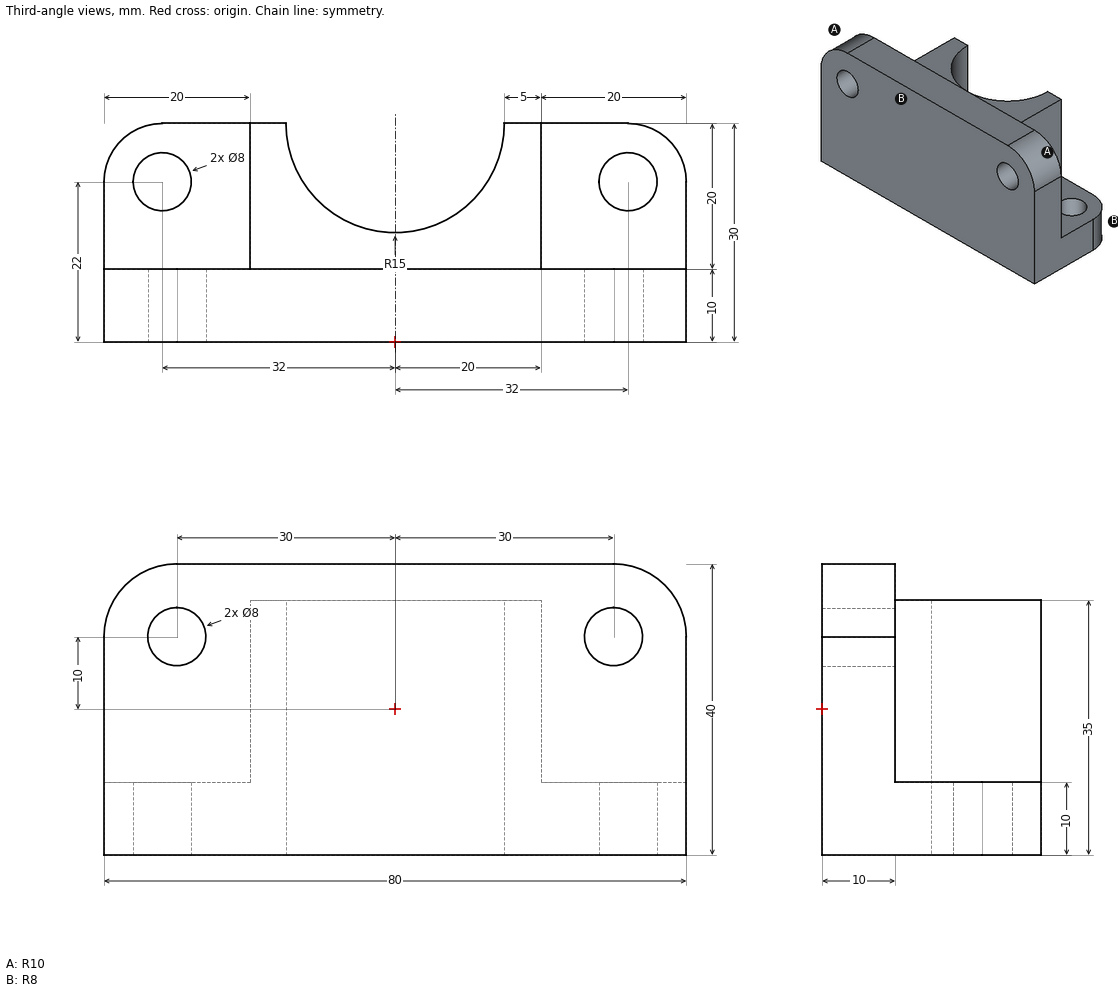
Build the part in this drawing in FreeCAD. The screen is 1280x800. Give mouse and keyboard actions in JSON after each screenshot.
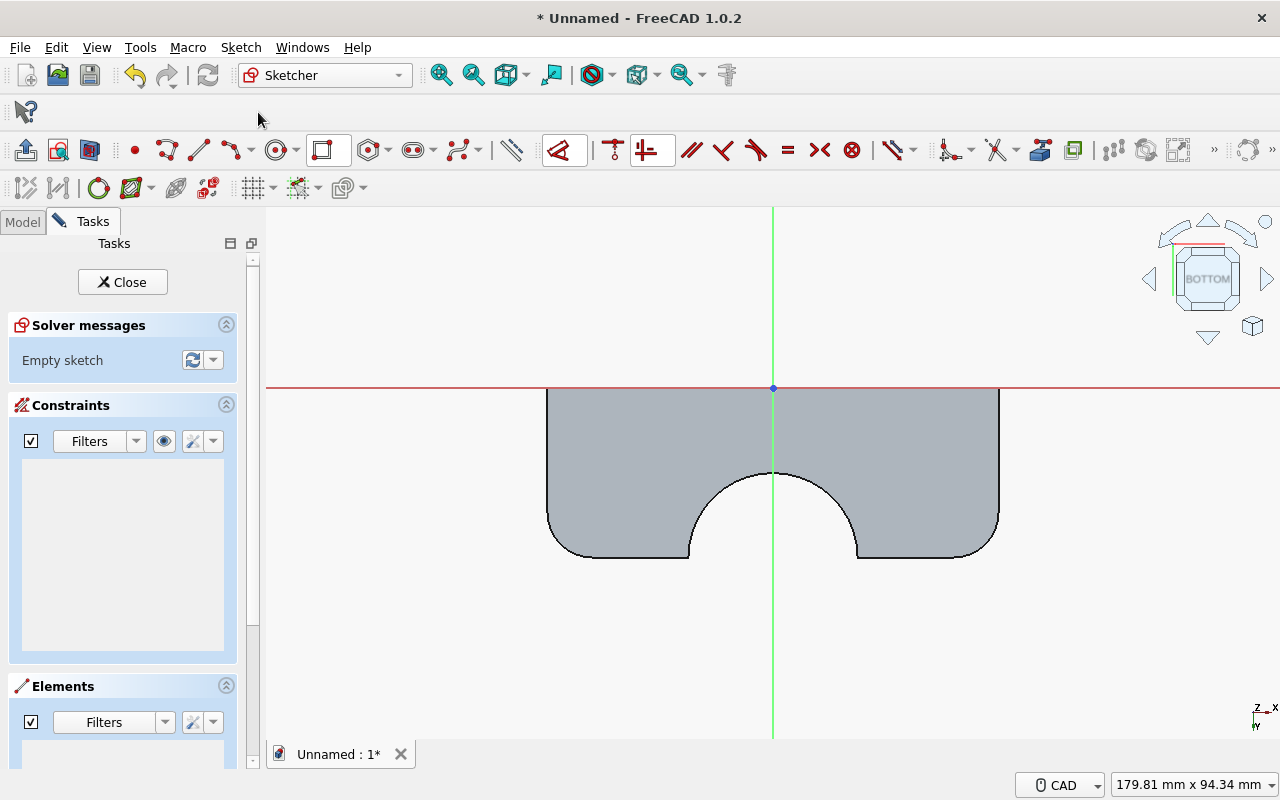
{"action": "scroll", "coordinate": [912, 439], "scroll_direction": "up", "scroll_amount": 2}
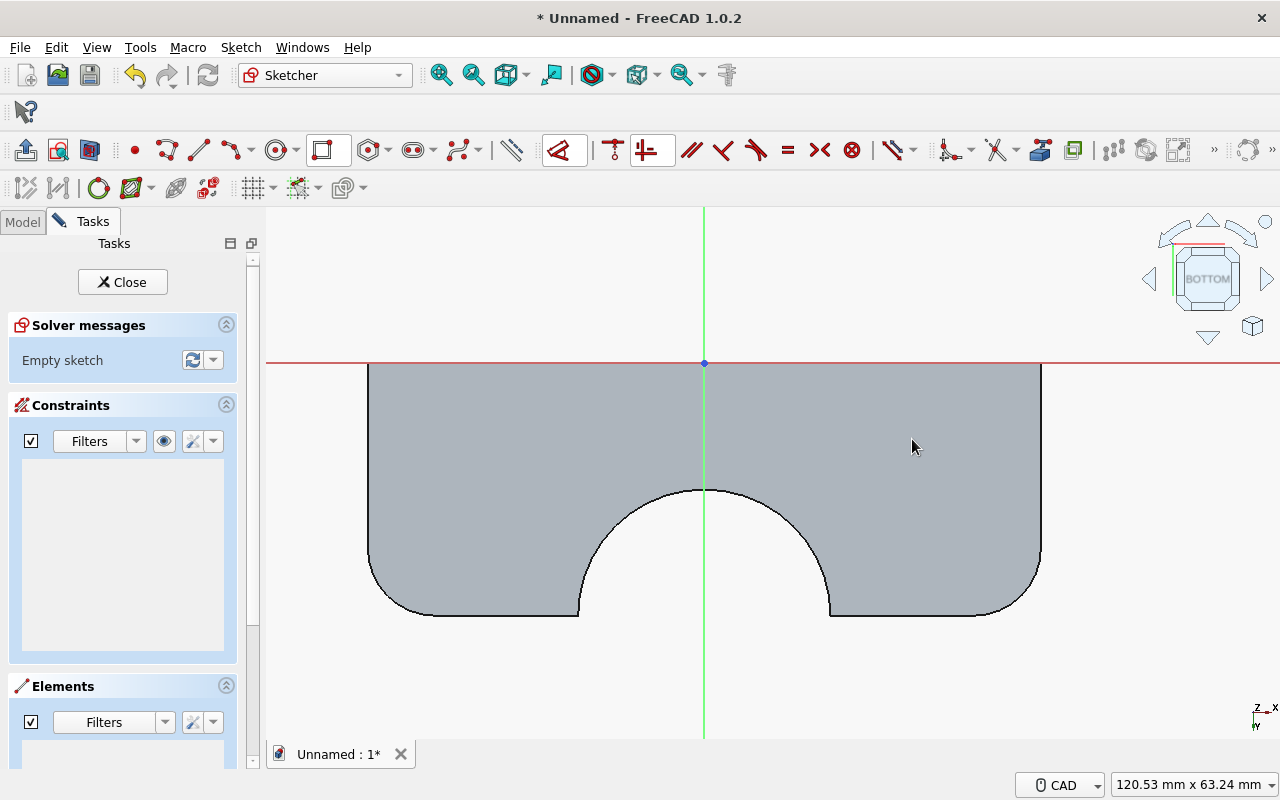
{"action": "left_click", "coordinate": [276, 150]}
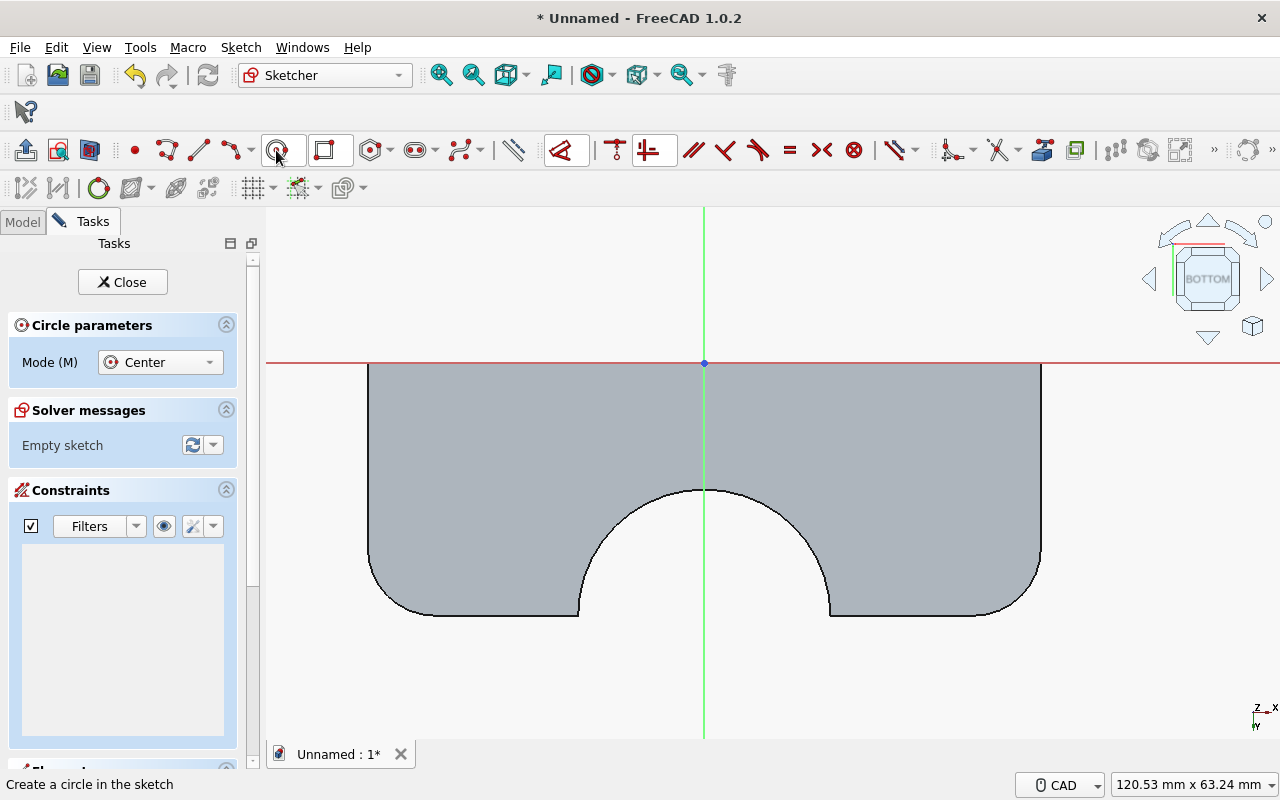
{"action": "left_click", "coordinate": [435, 548]}
{"action": "mouse_move", "coordinate": [459, 525]}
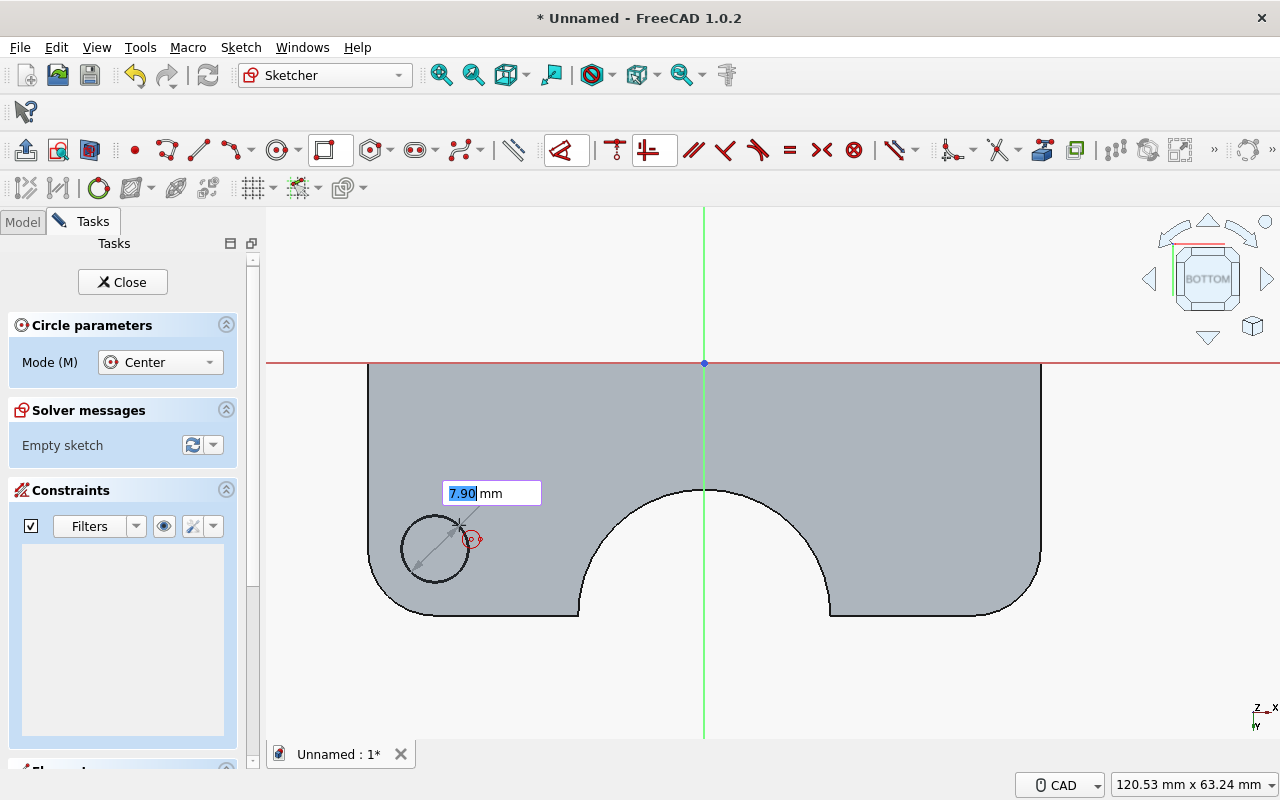
{"action": "type", "text": "8"}
{"action": "key", "text": "Return"}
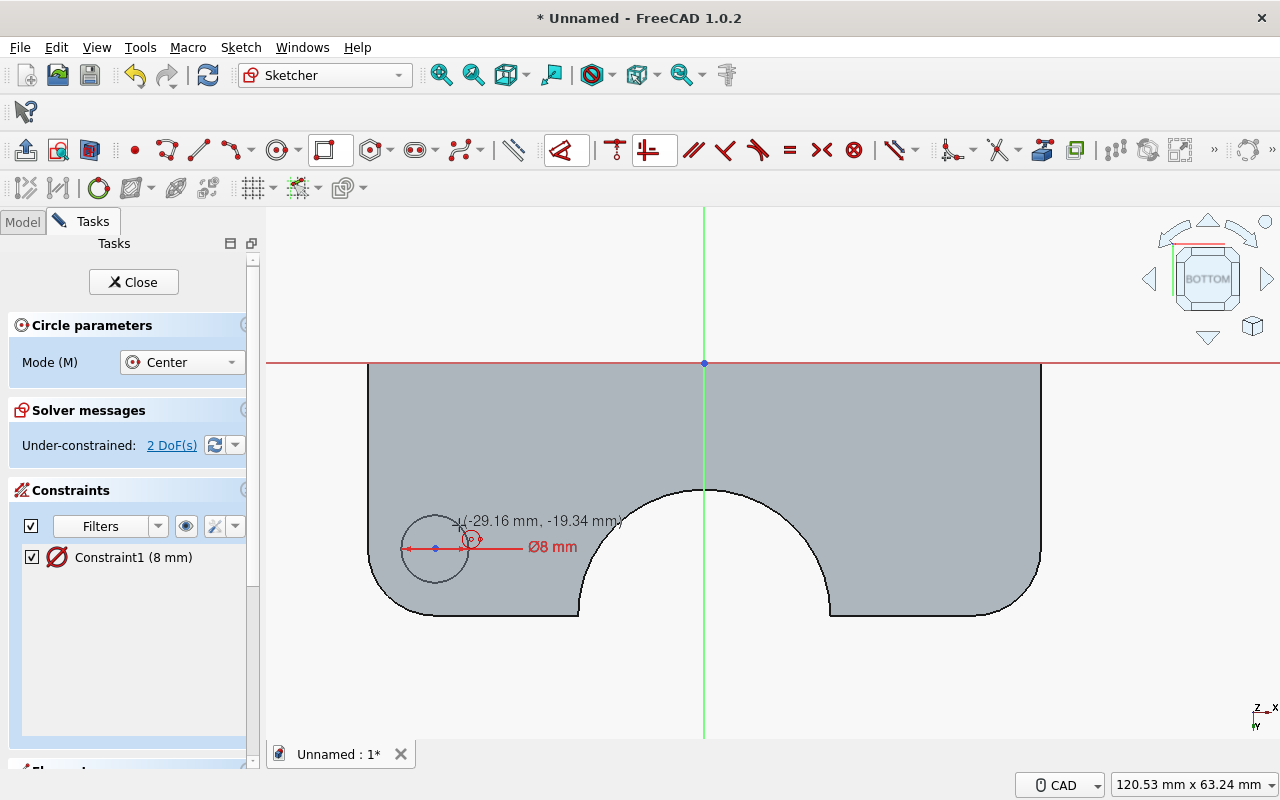
{"action": "left_click", "coordinate": [974, 548]}
{"action": "mouse_move", "coordinate": [997, 525]}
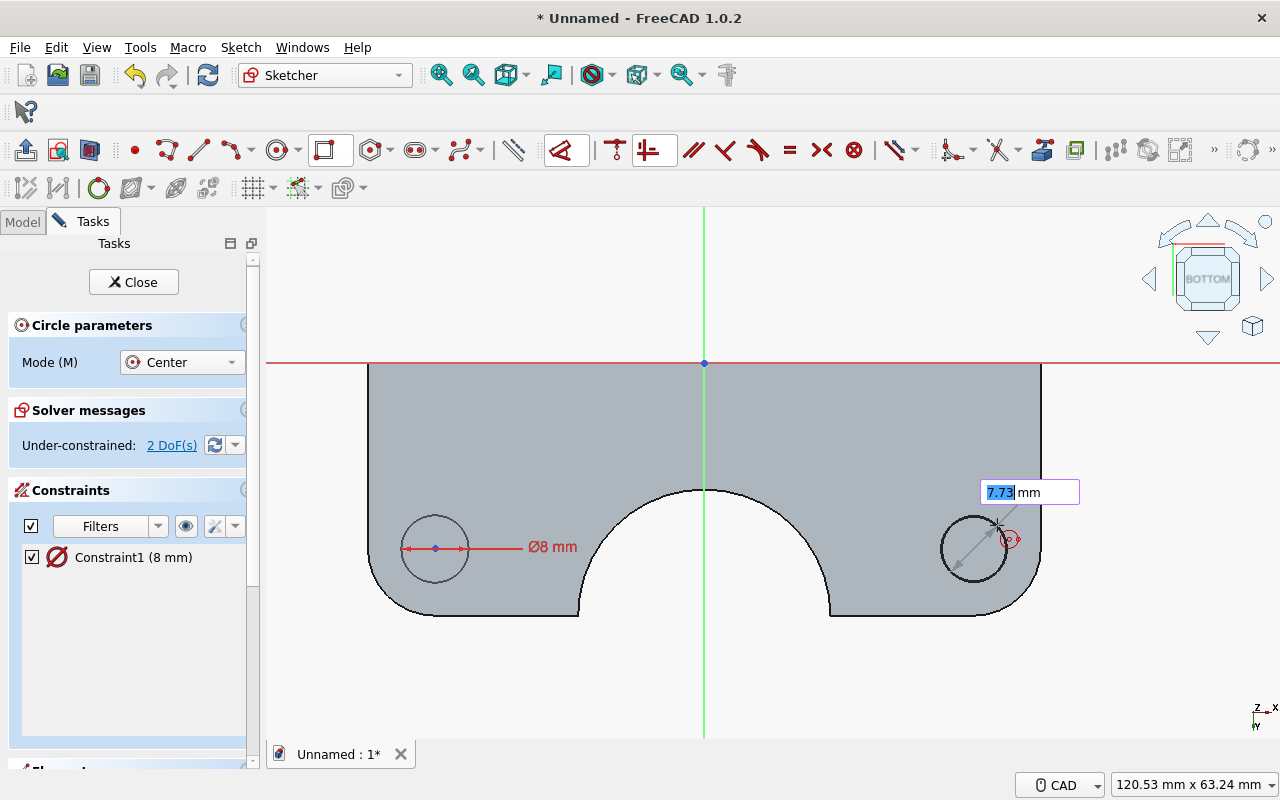
{"action": "type", "text": "8"}
{"action": "key", "text": "Return"}
{"action": "key", "text": "Escape"}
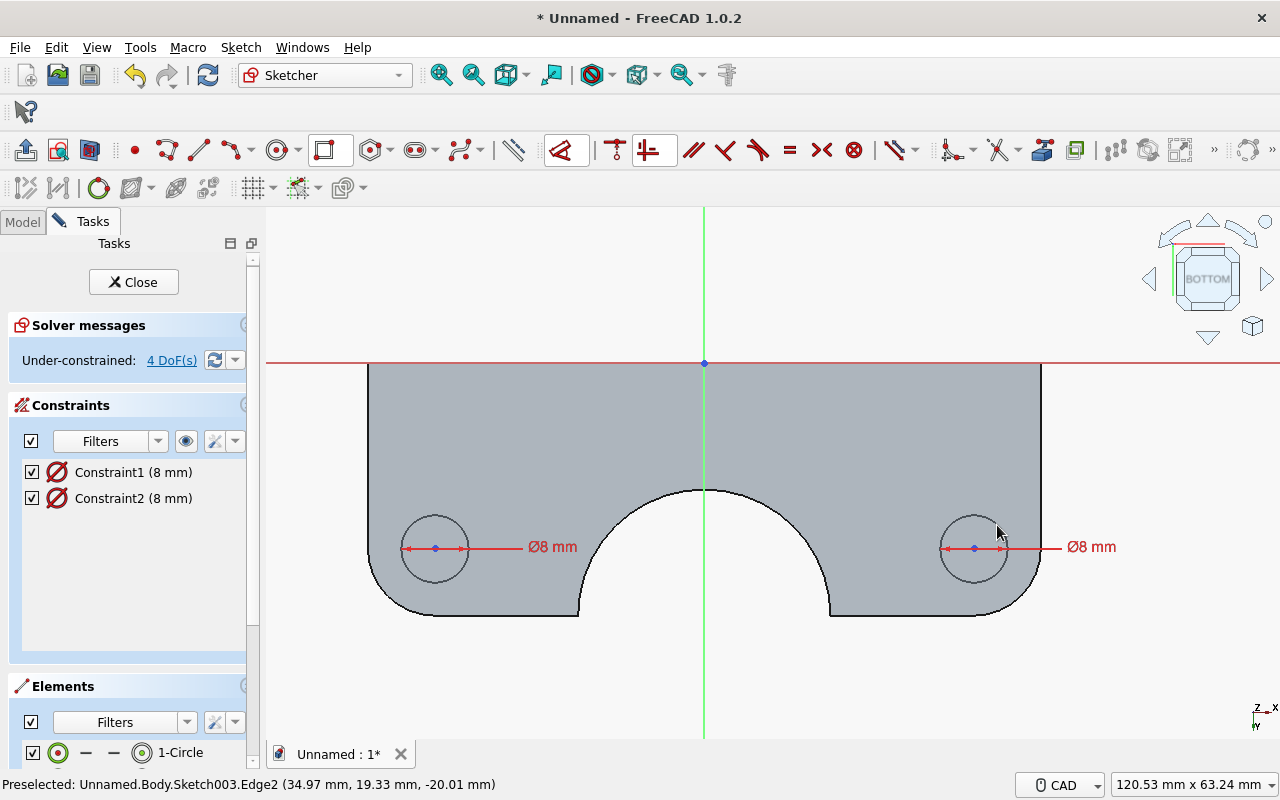
{"action": "left_click", "coordinate": [435, 549]}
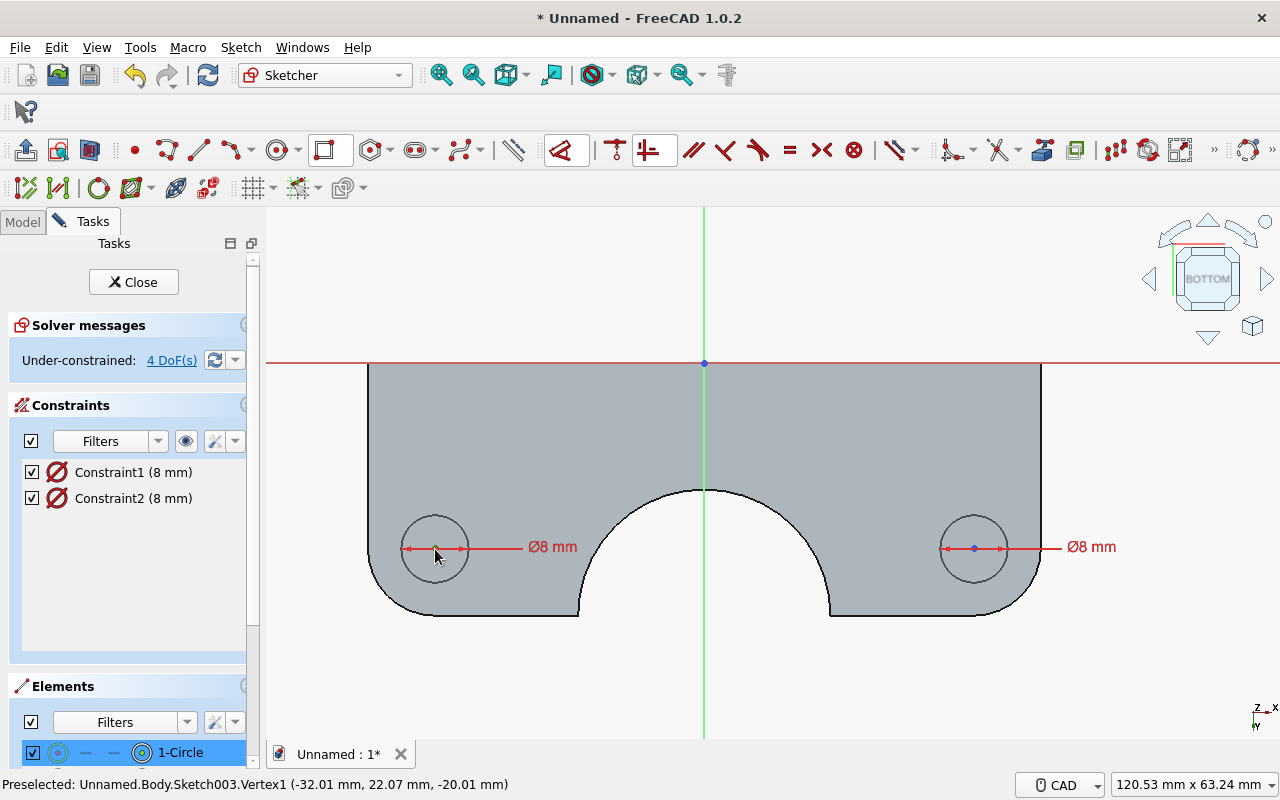
{"action": "left_click", "coordinate": [974, 549]}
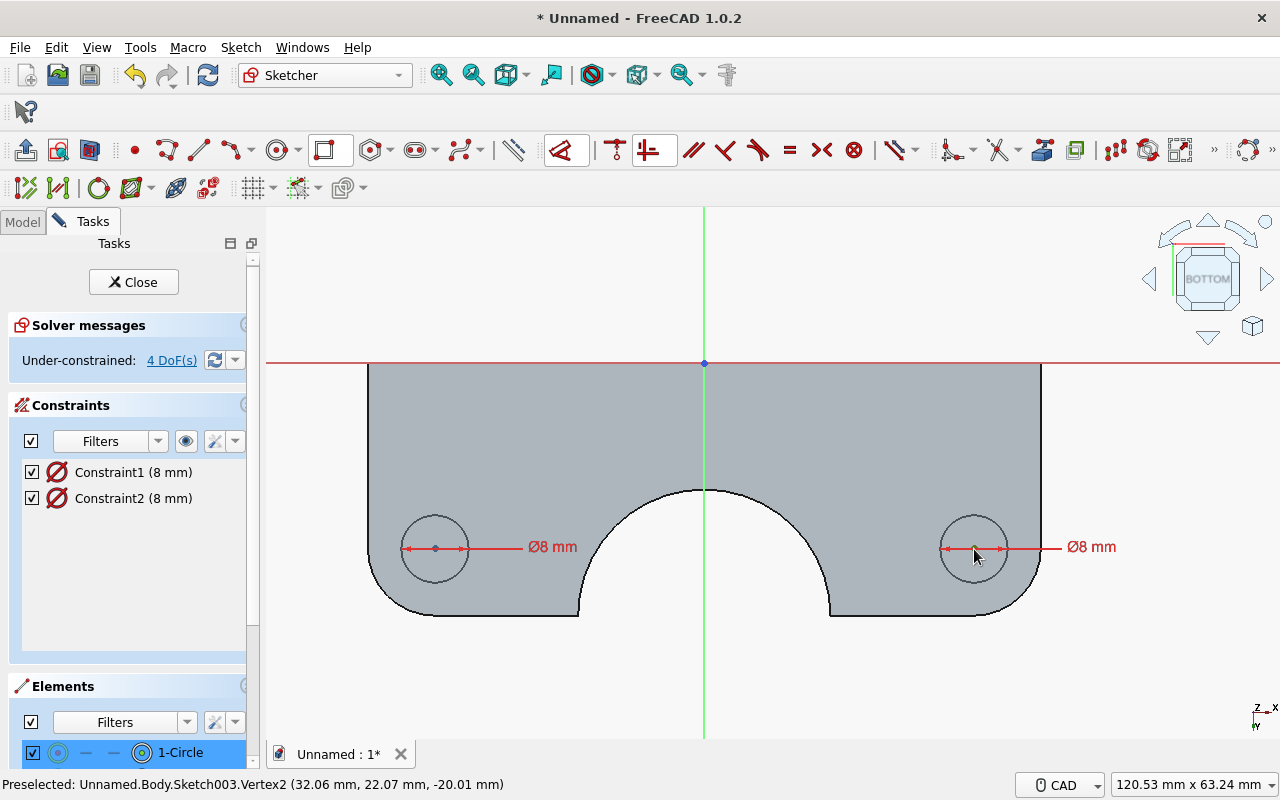
{"action": "key", "text": "h"}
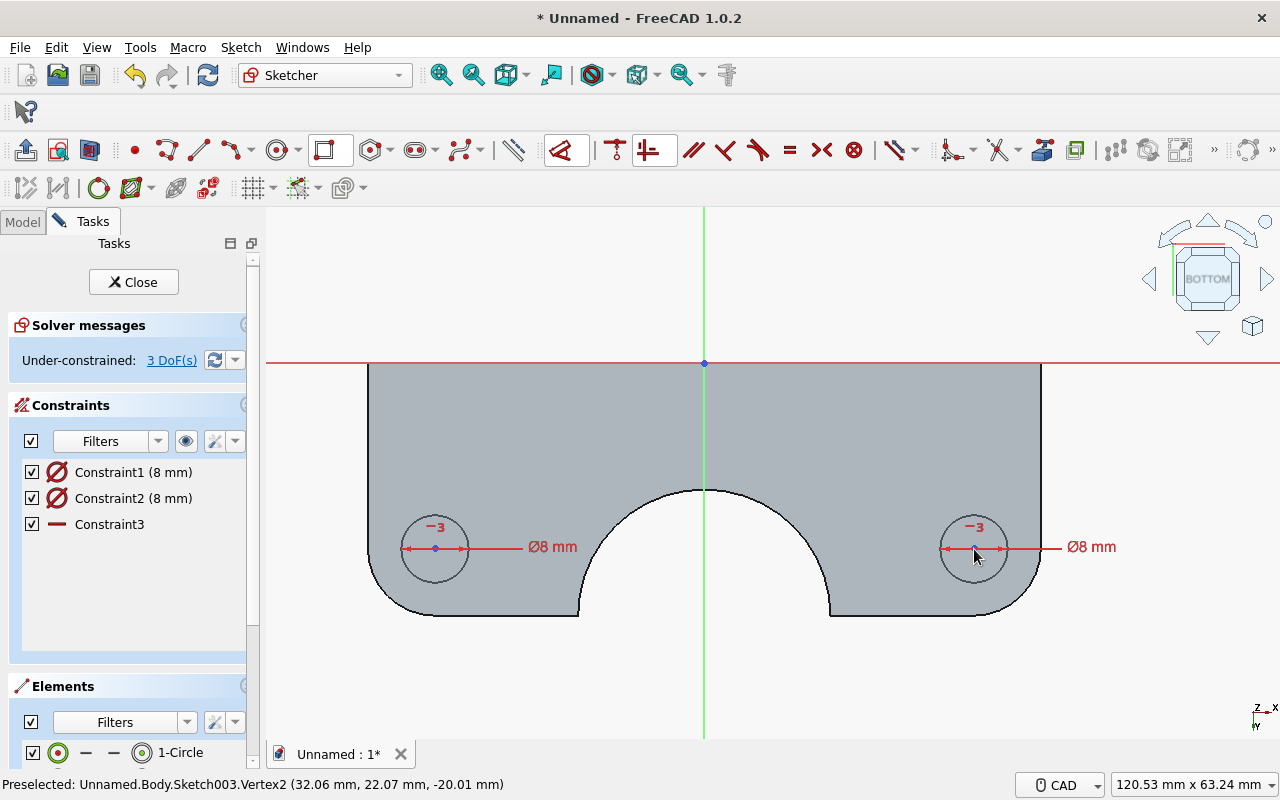
{"action": "left_click", "coordinate": [435, 549]}